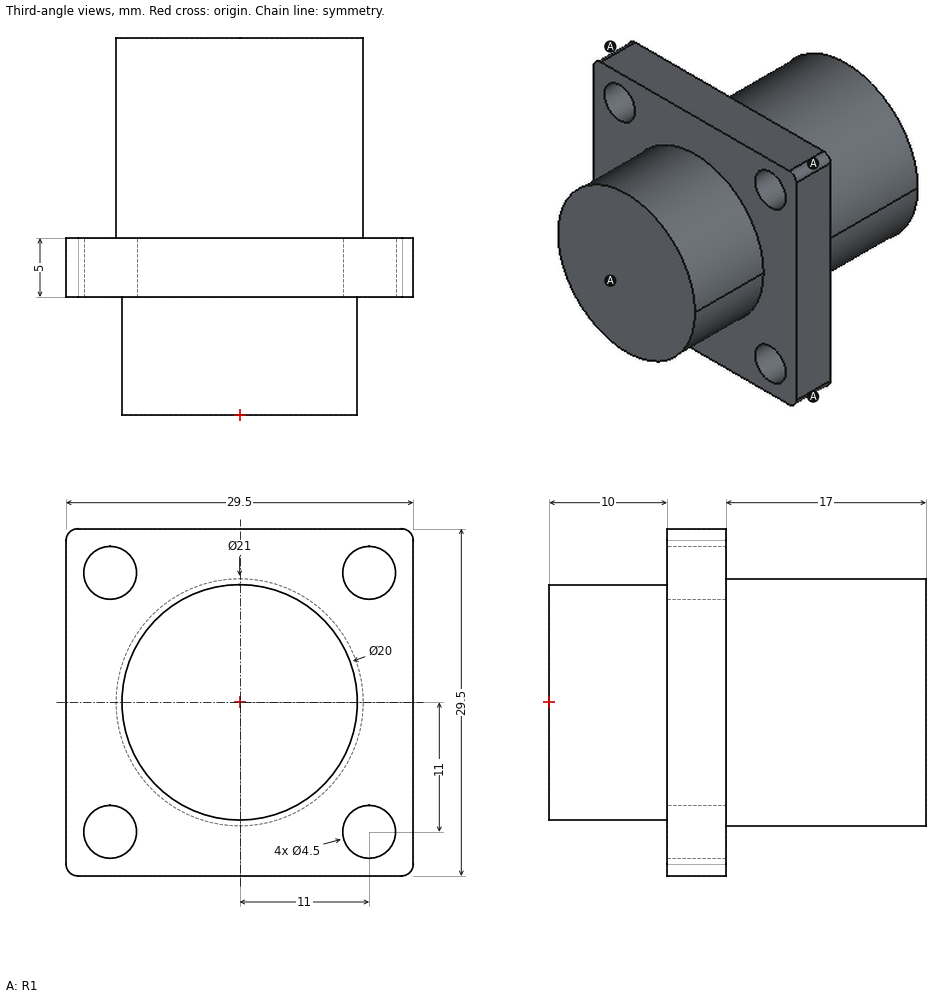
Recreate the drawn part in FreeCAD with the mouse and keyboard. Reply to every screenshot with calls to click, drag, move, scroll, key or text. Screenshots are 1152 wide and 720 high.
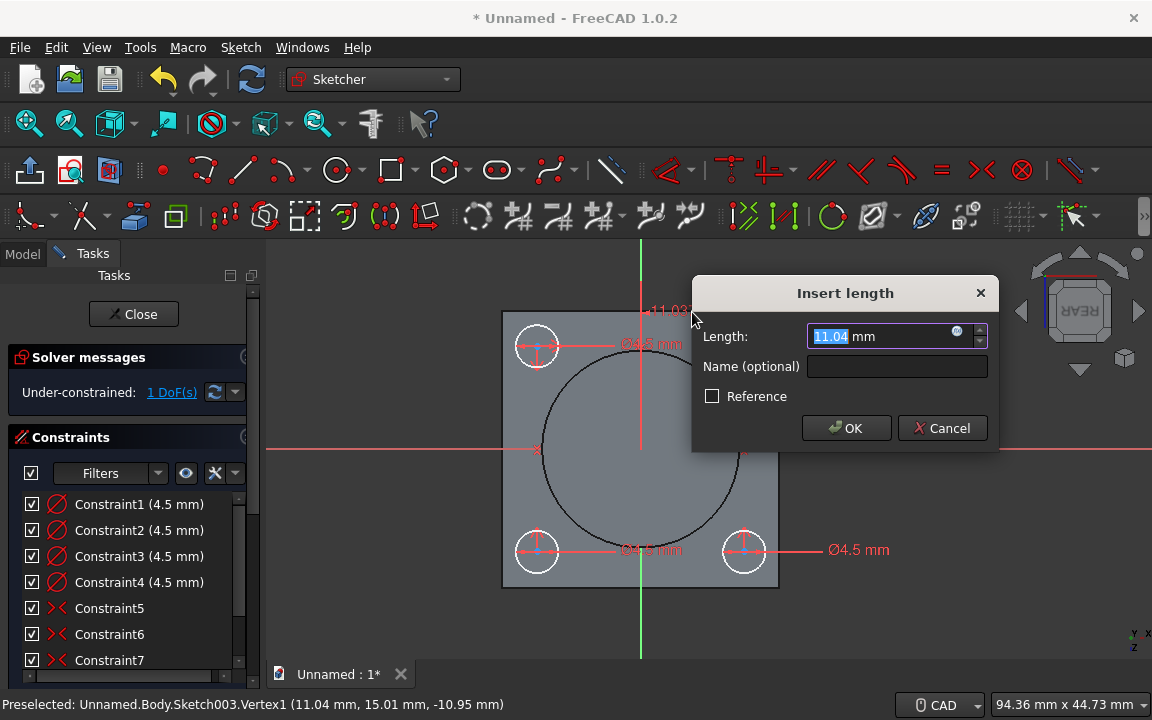
text(11)
key(Return)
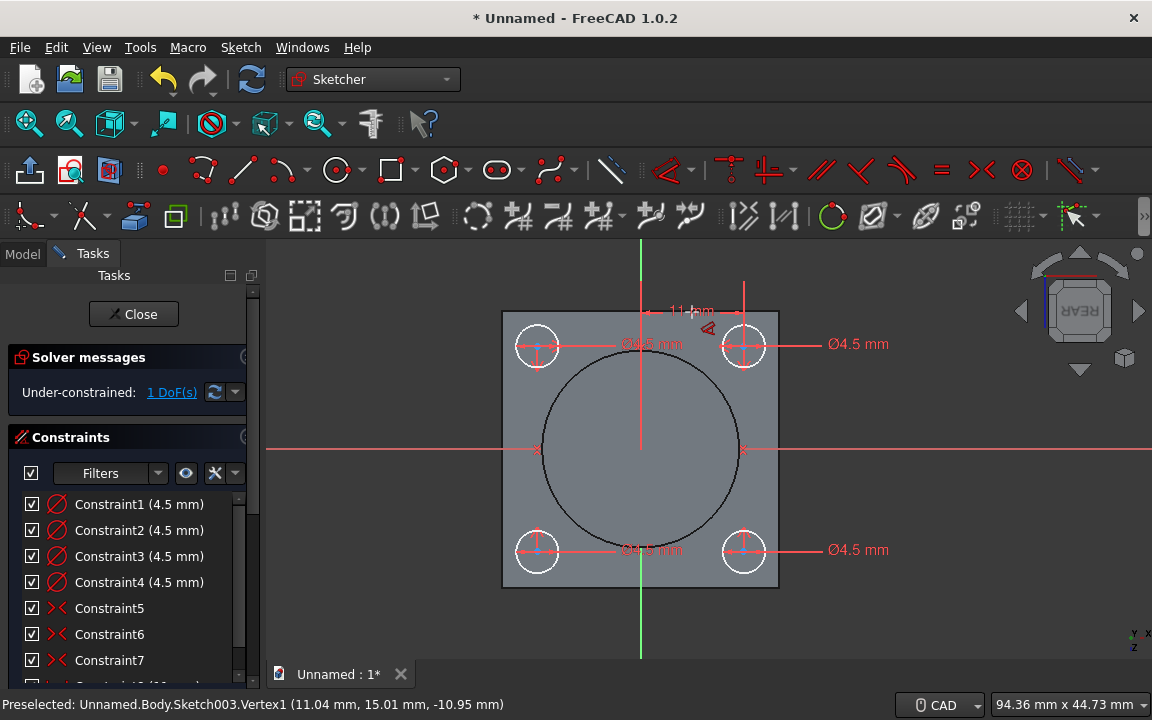
click(744, 346)
click(778, 398)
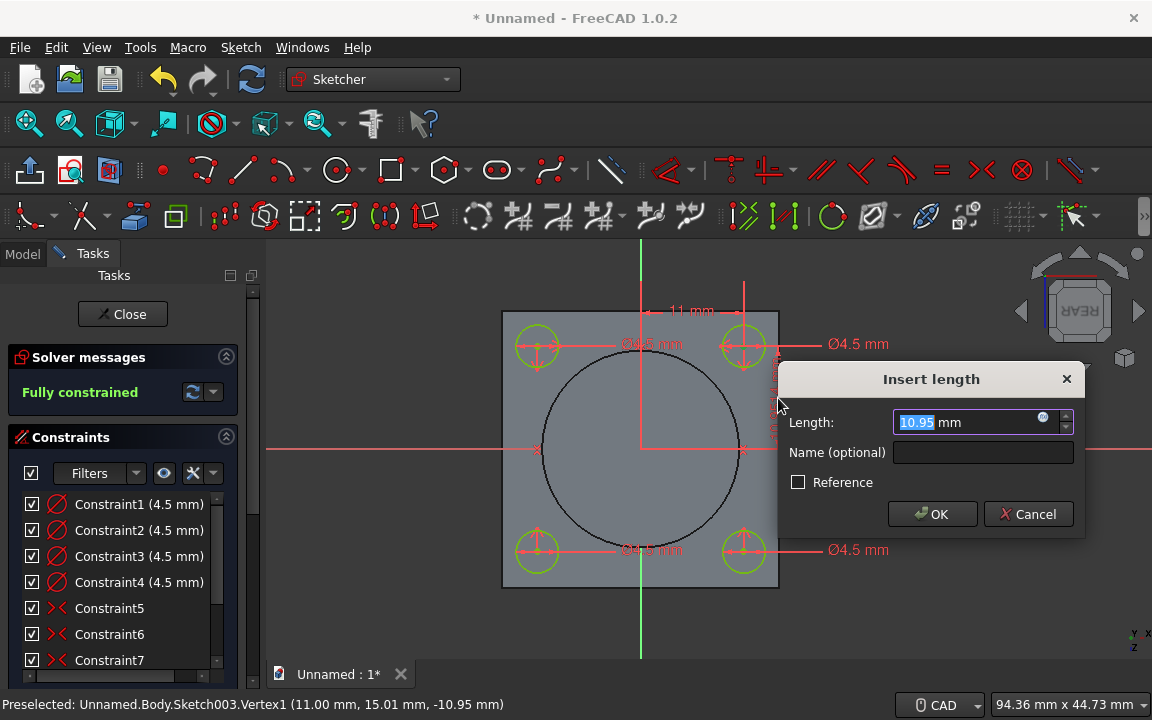
text(11)
key(Return)
key(Escape)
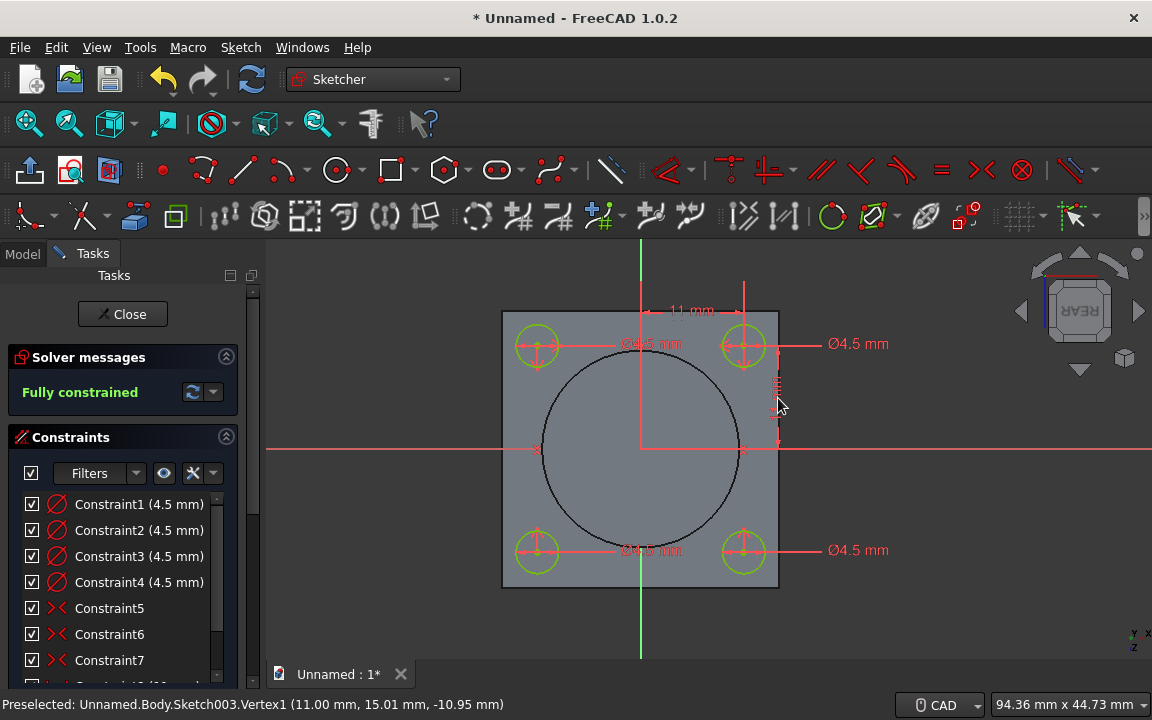
click(123, 314)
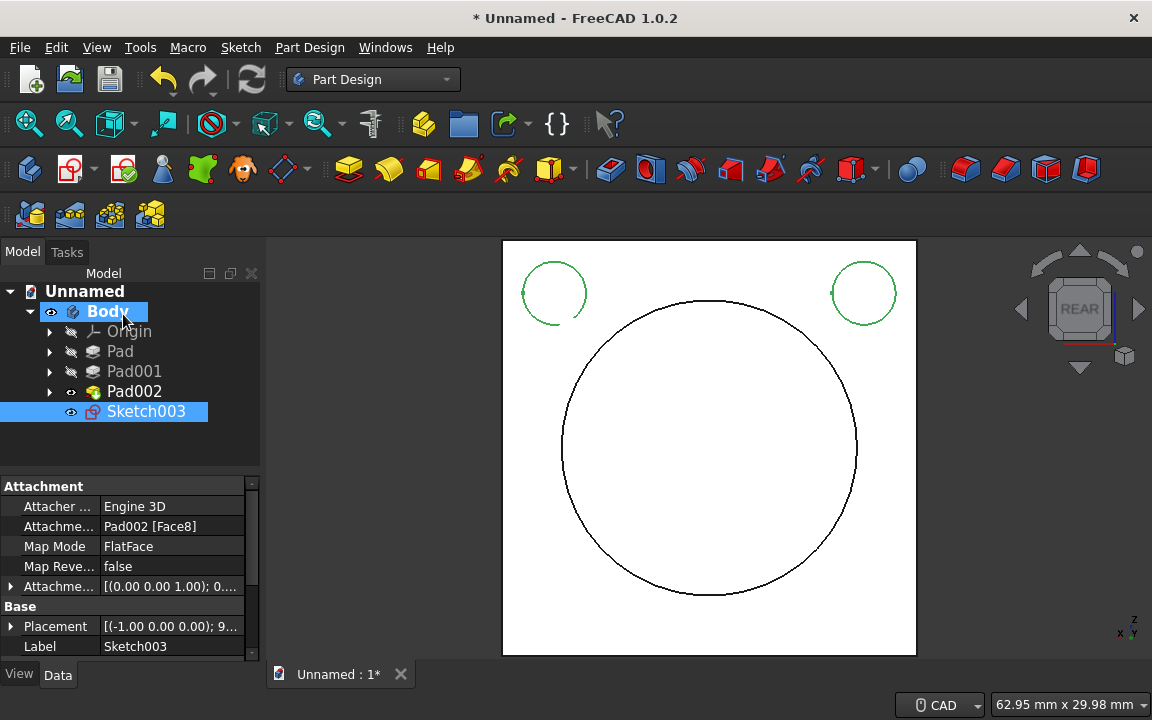
click(612, 170)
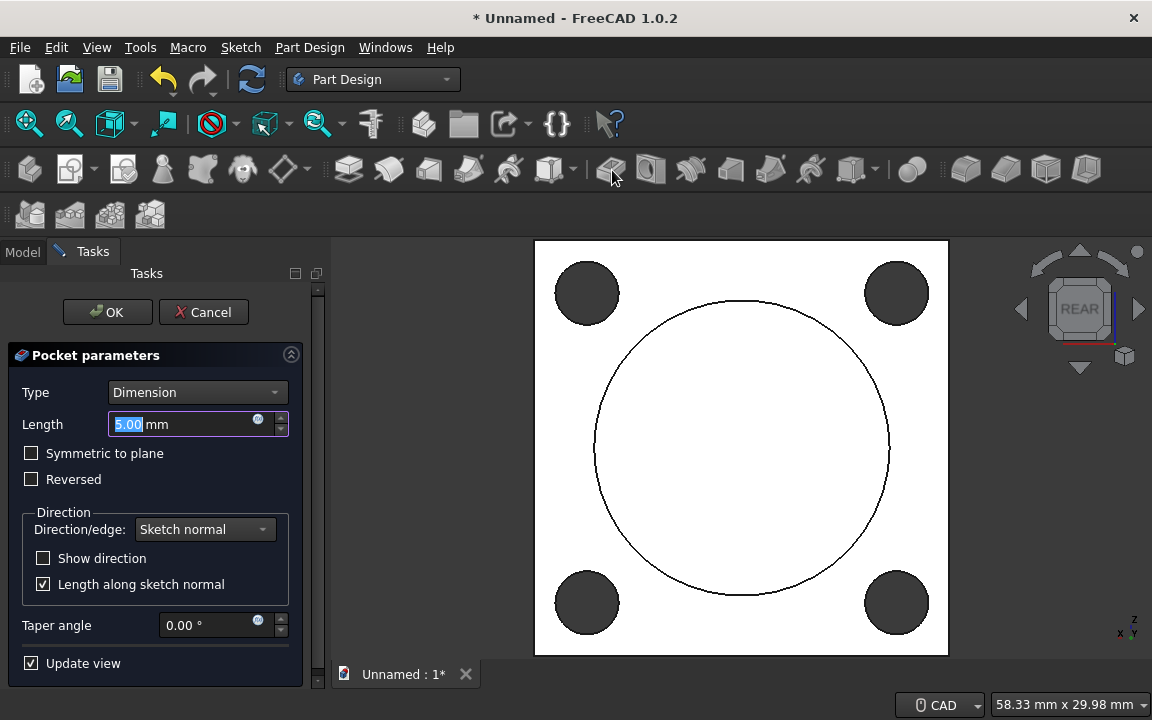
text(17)
key(Tab)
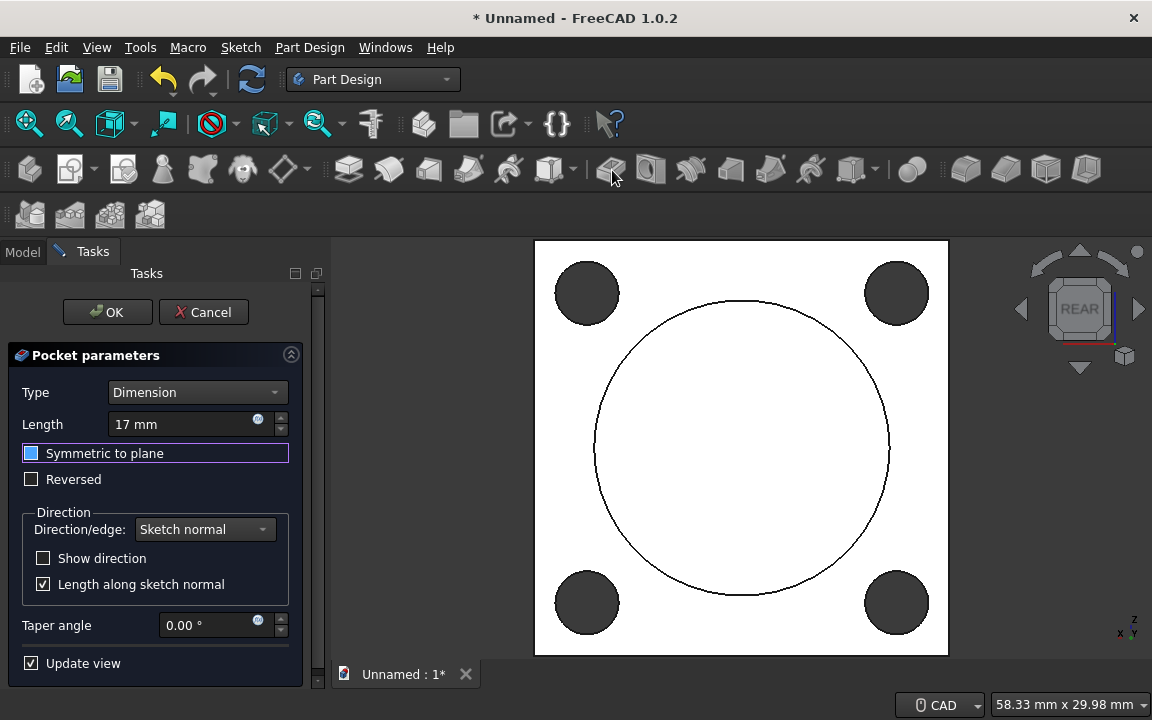
click(108, 312)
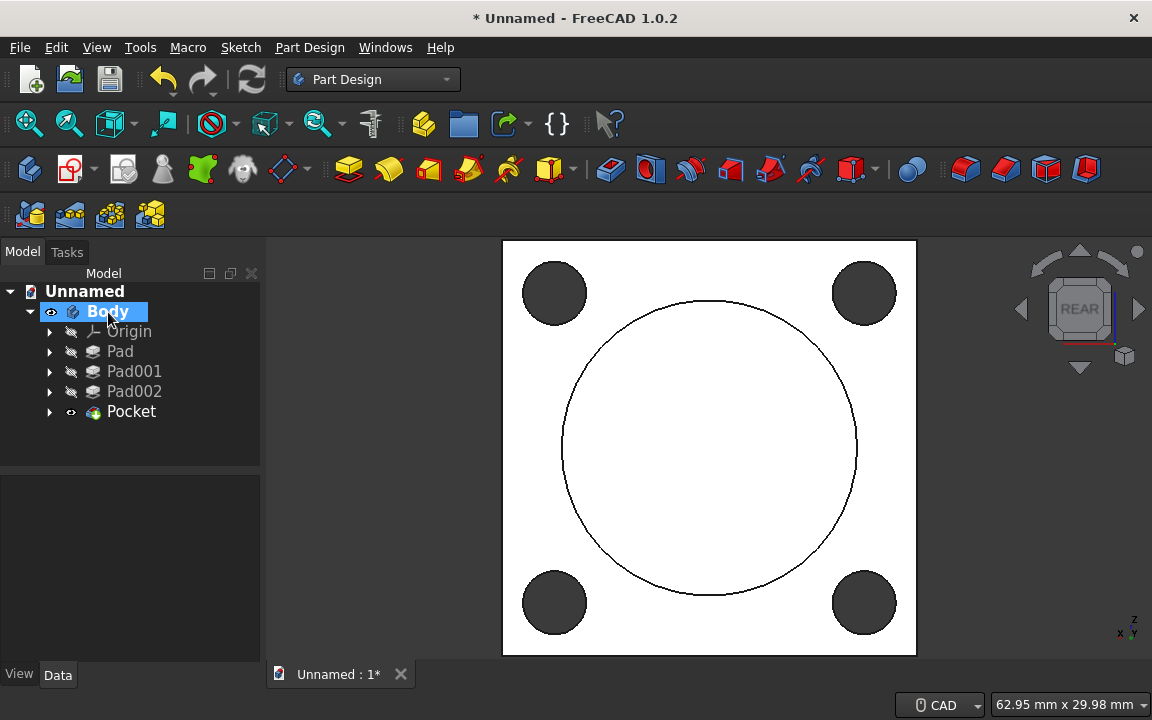
key(0)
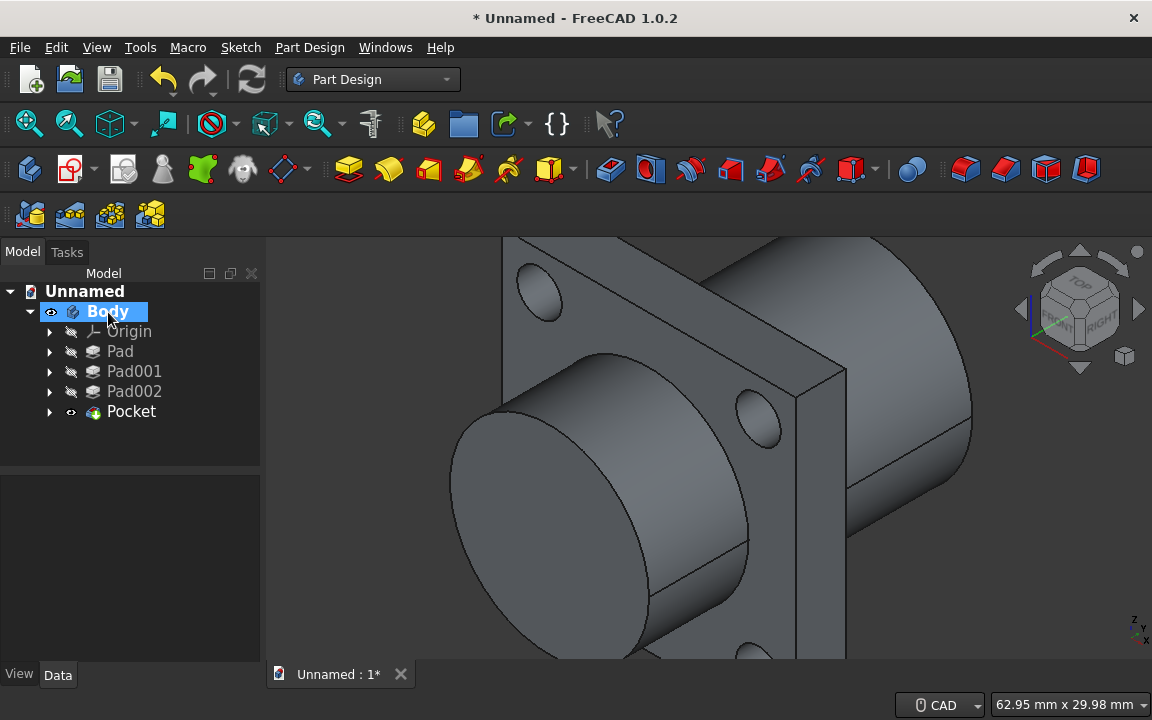
key(v)
key(f)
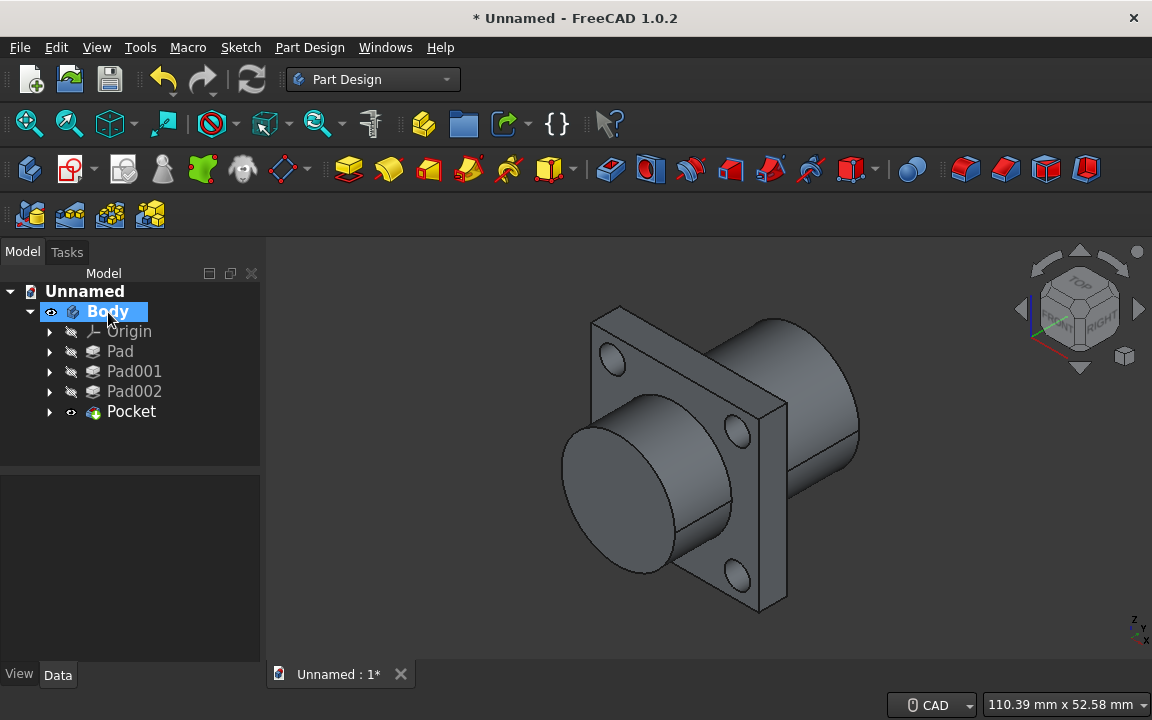
click(773, 410)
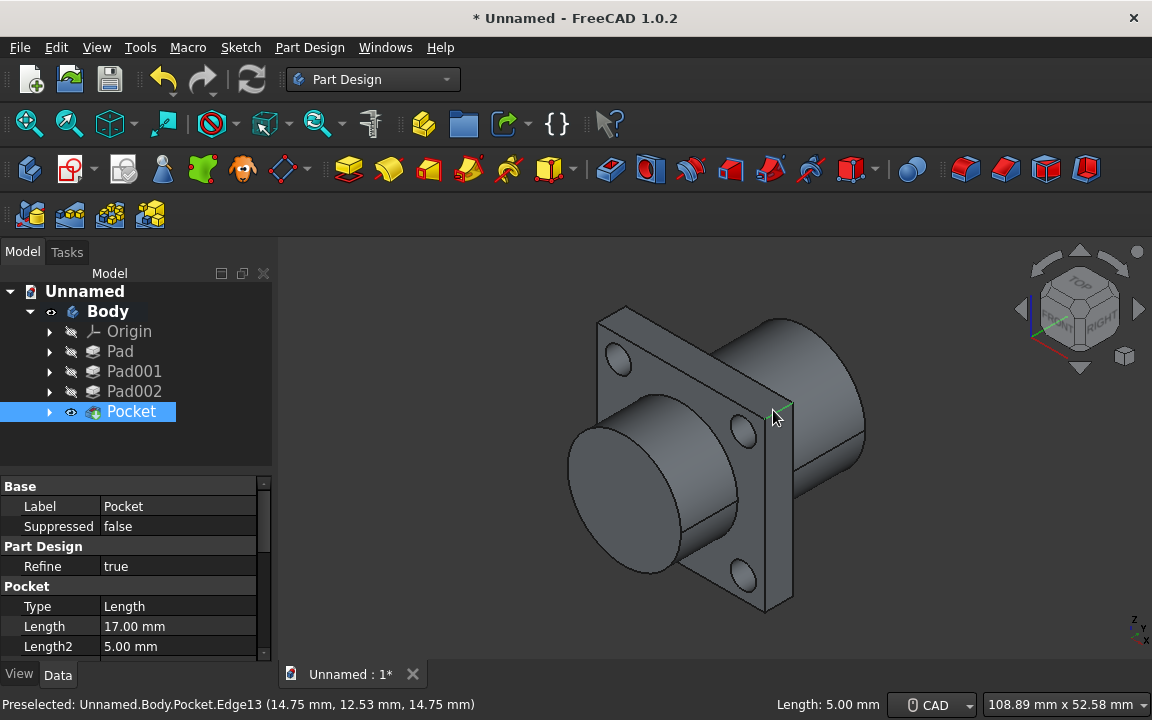
key(2)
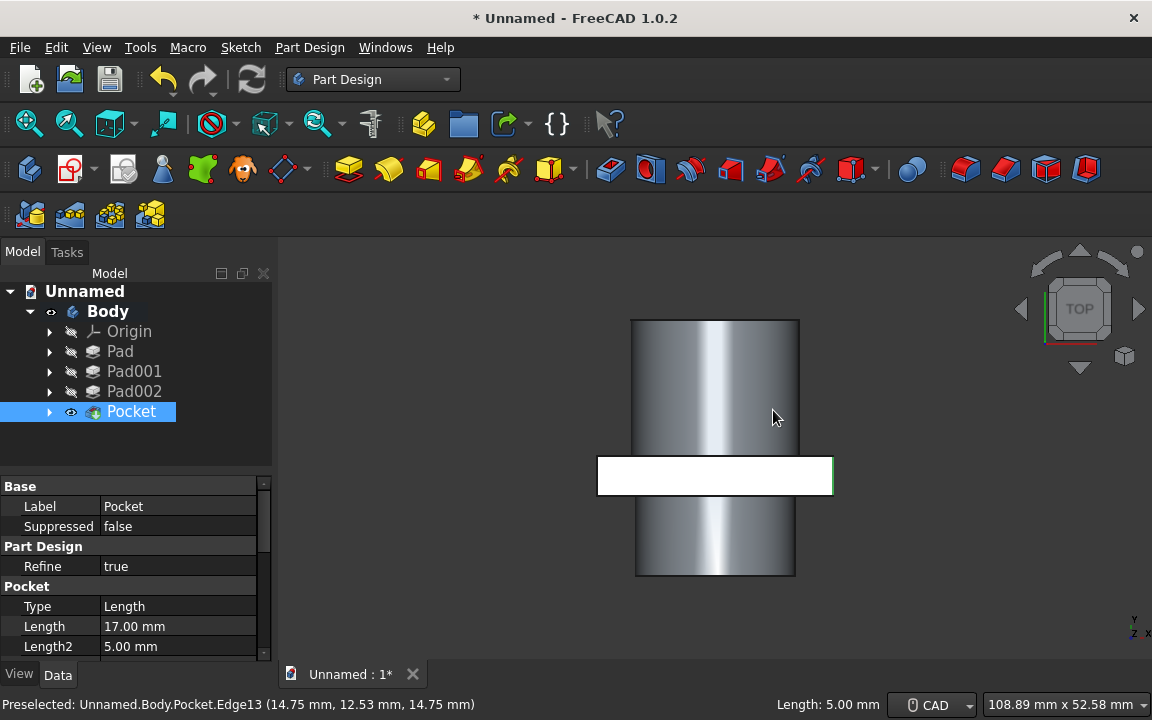
click(597, 475, ctrl)